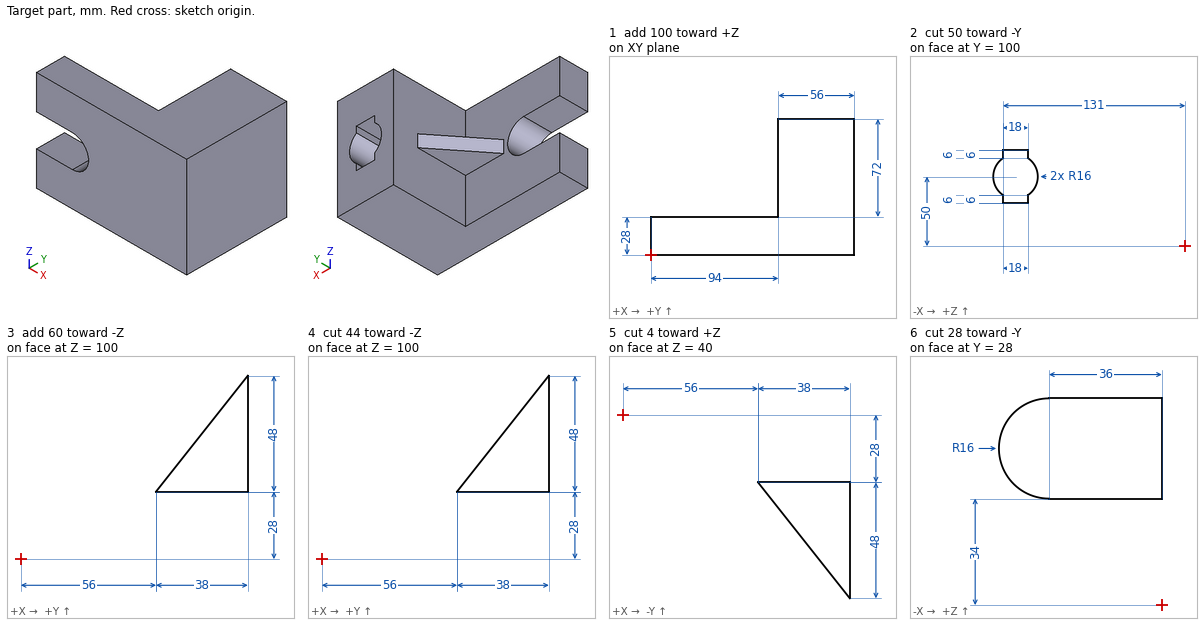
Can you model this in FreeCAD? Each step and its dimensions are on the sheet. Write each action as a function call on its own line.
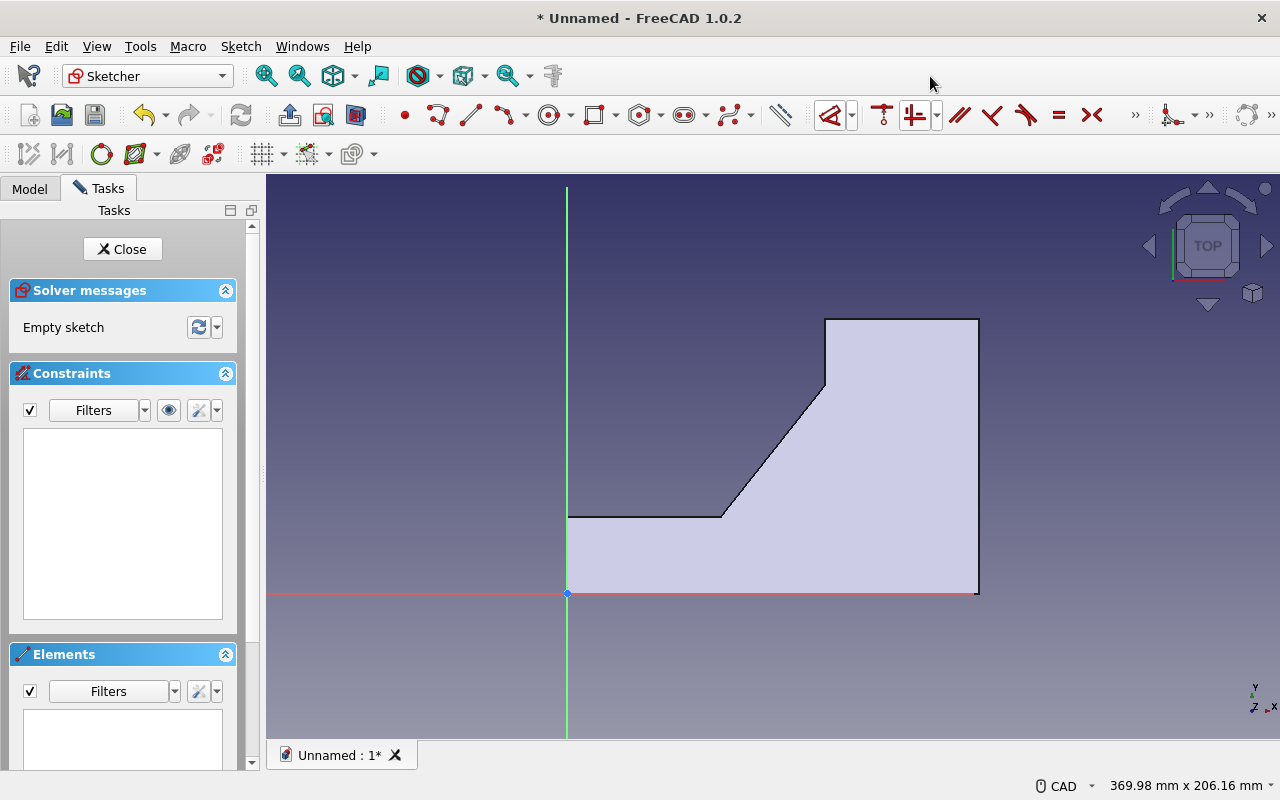
scroll(686, 529, up, 3)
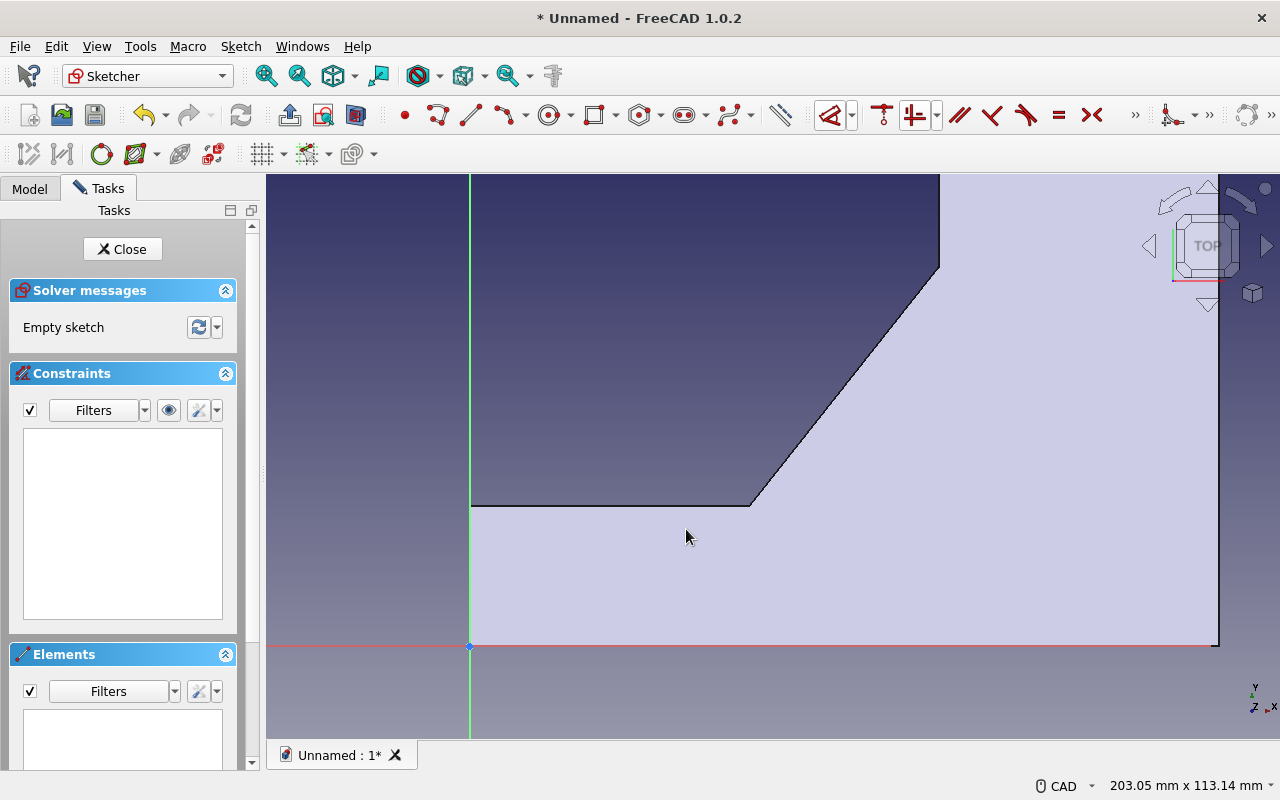
click(438, 116)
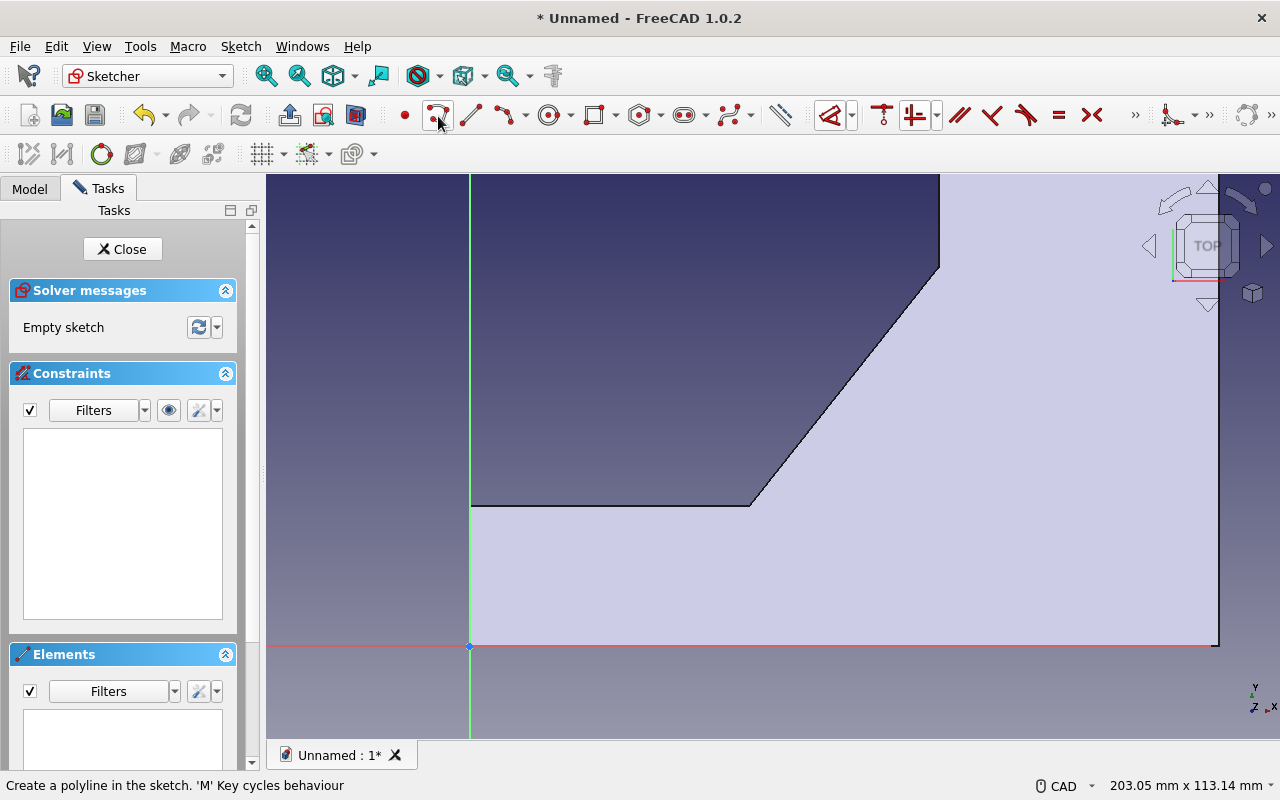
click(749, 506)
click(939, 506)
click(939, 267)
click(749, 507)
key(Escape)
key(Escape)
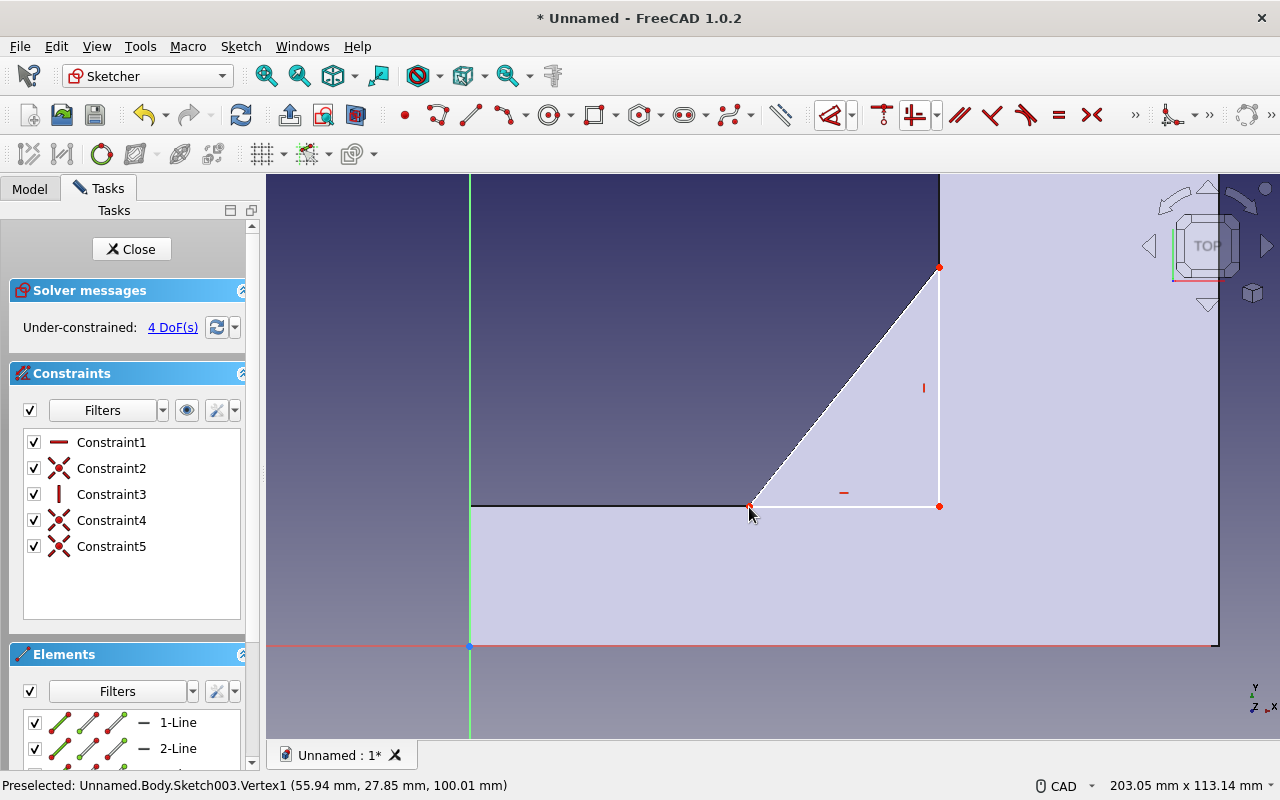
click(806, 507)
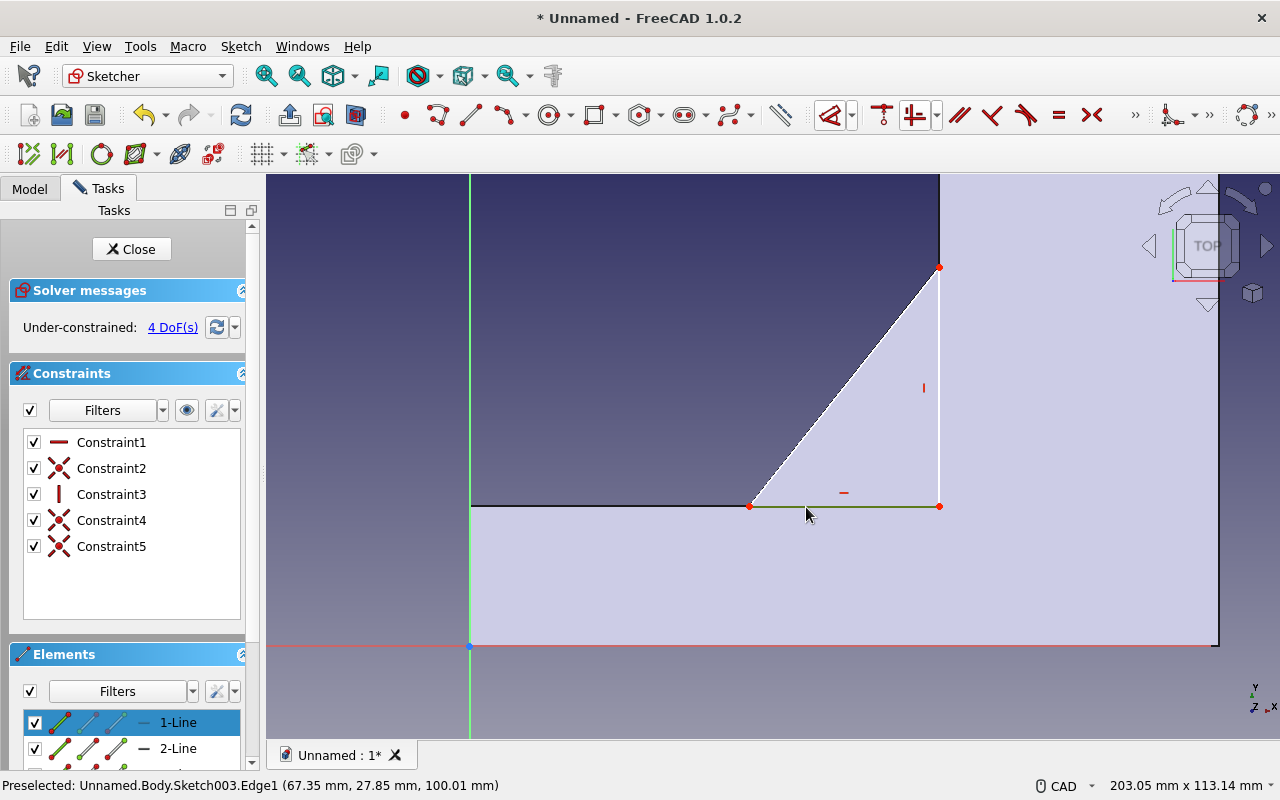
key(l)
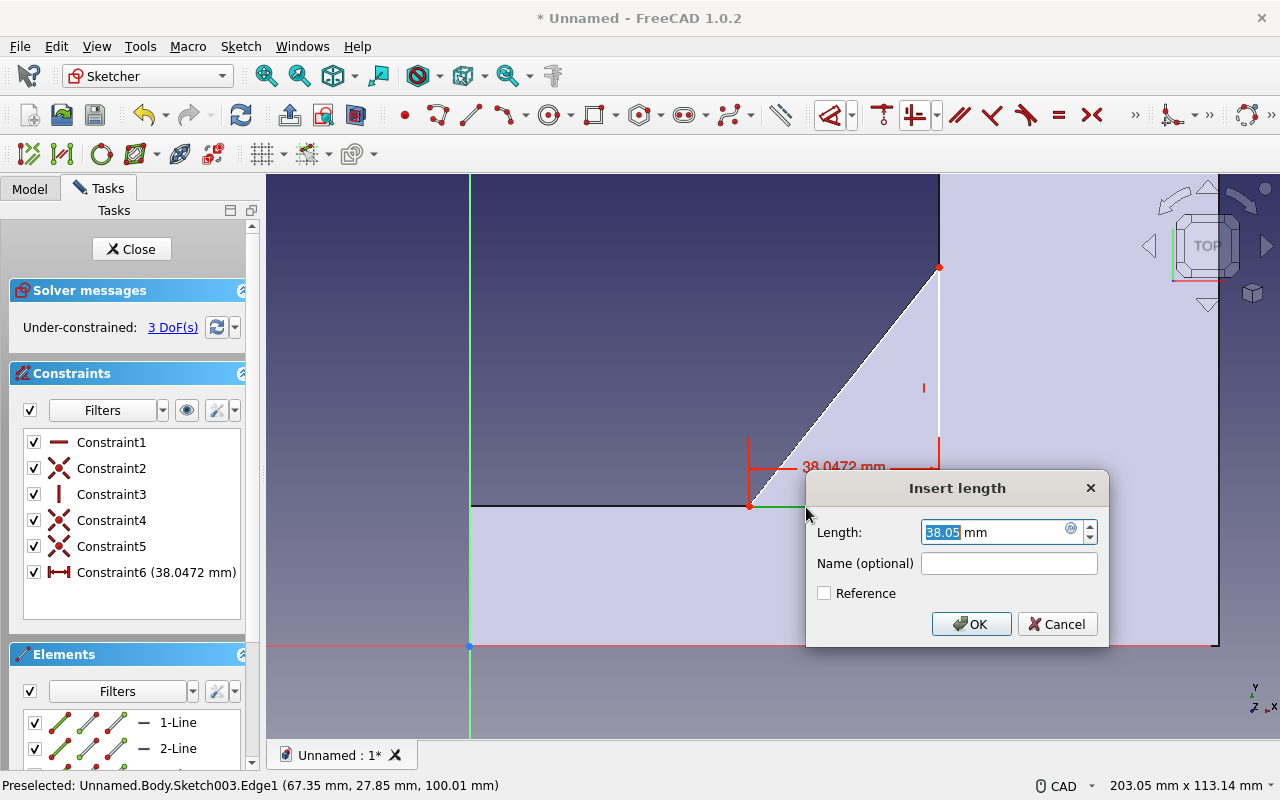
text(38)
key(Return)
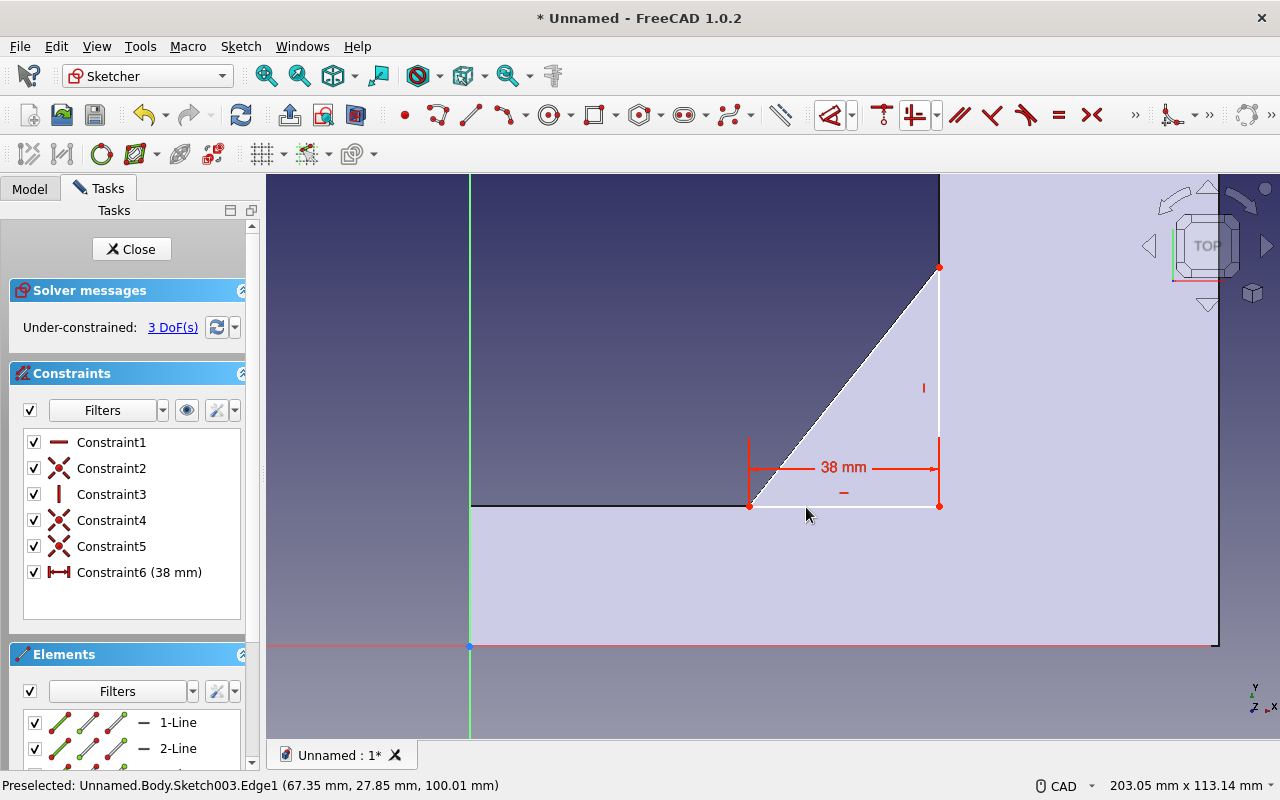
click(939, 435)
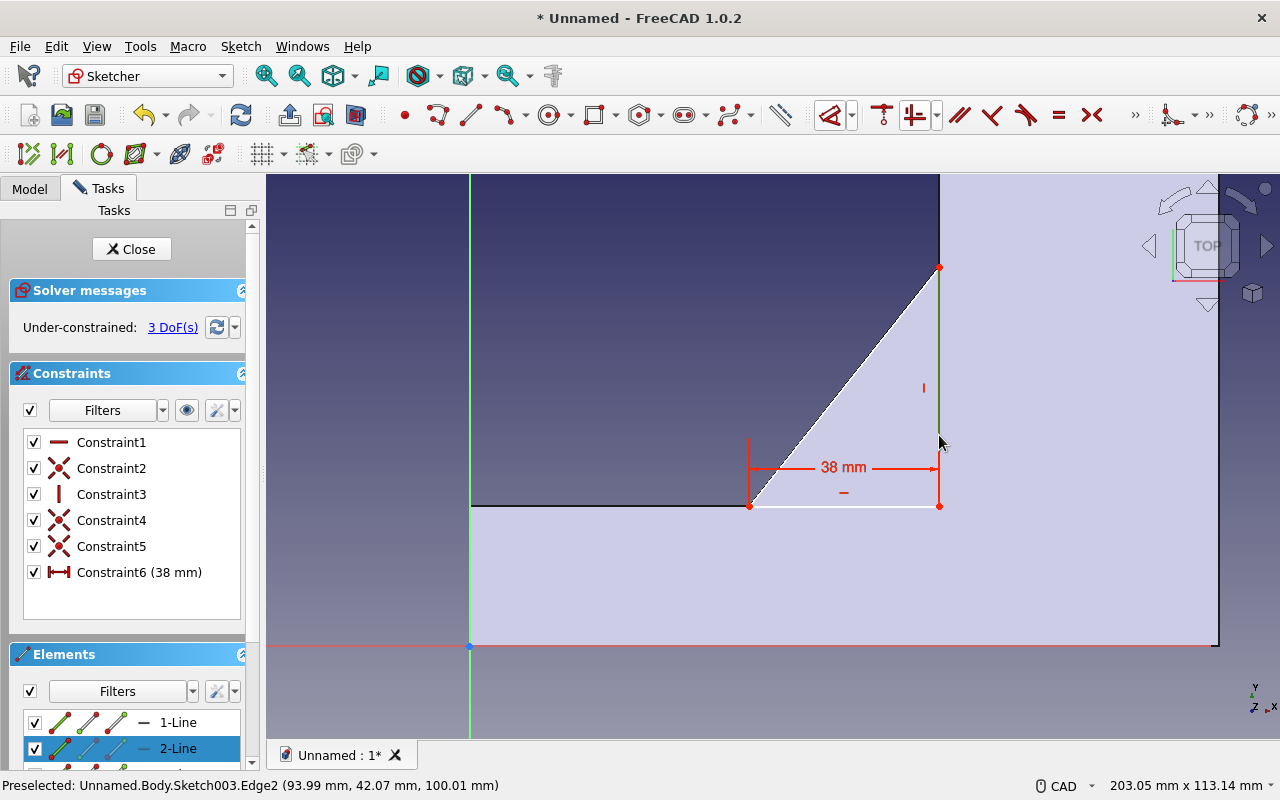
click(852, 116)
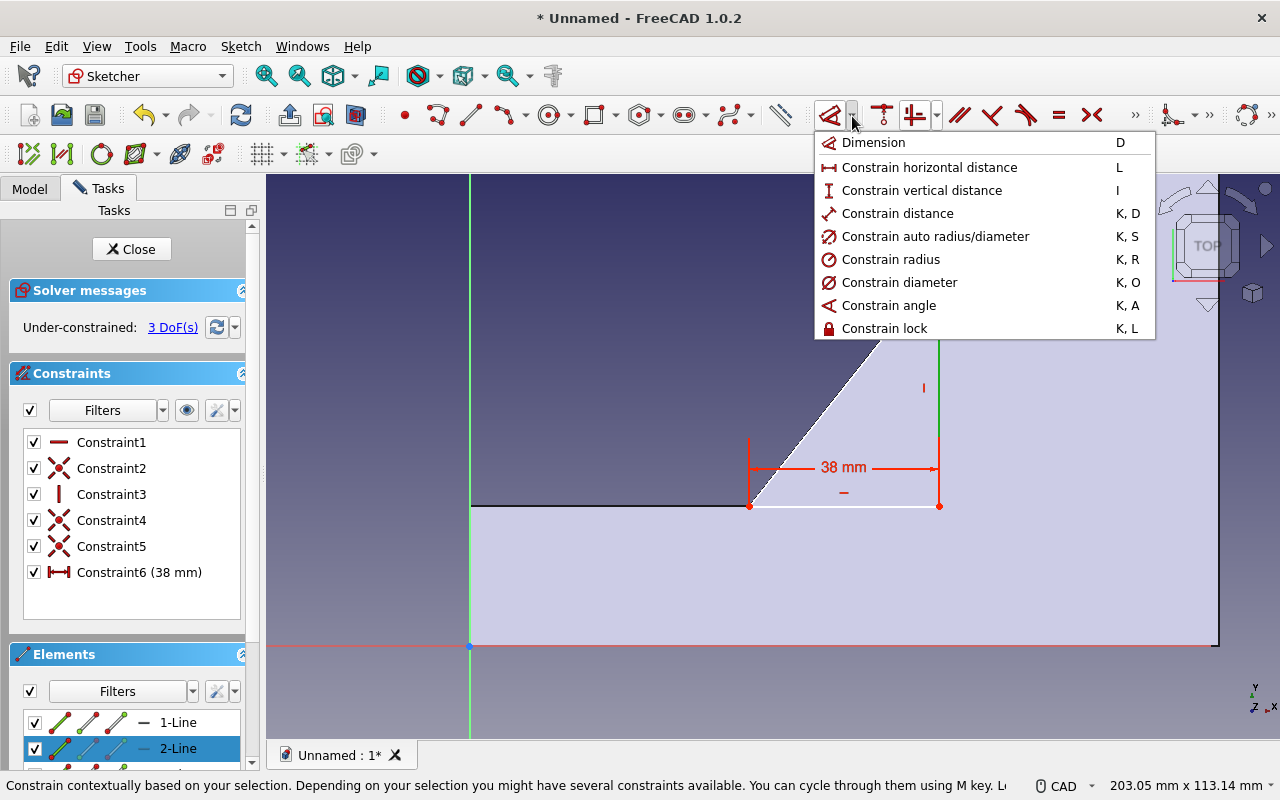
click(985, 190)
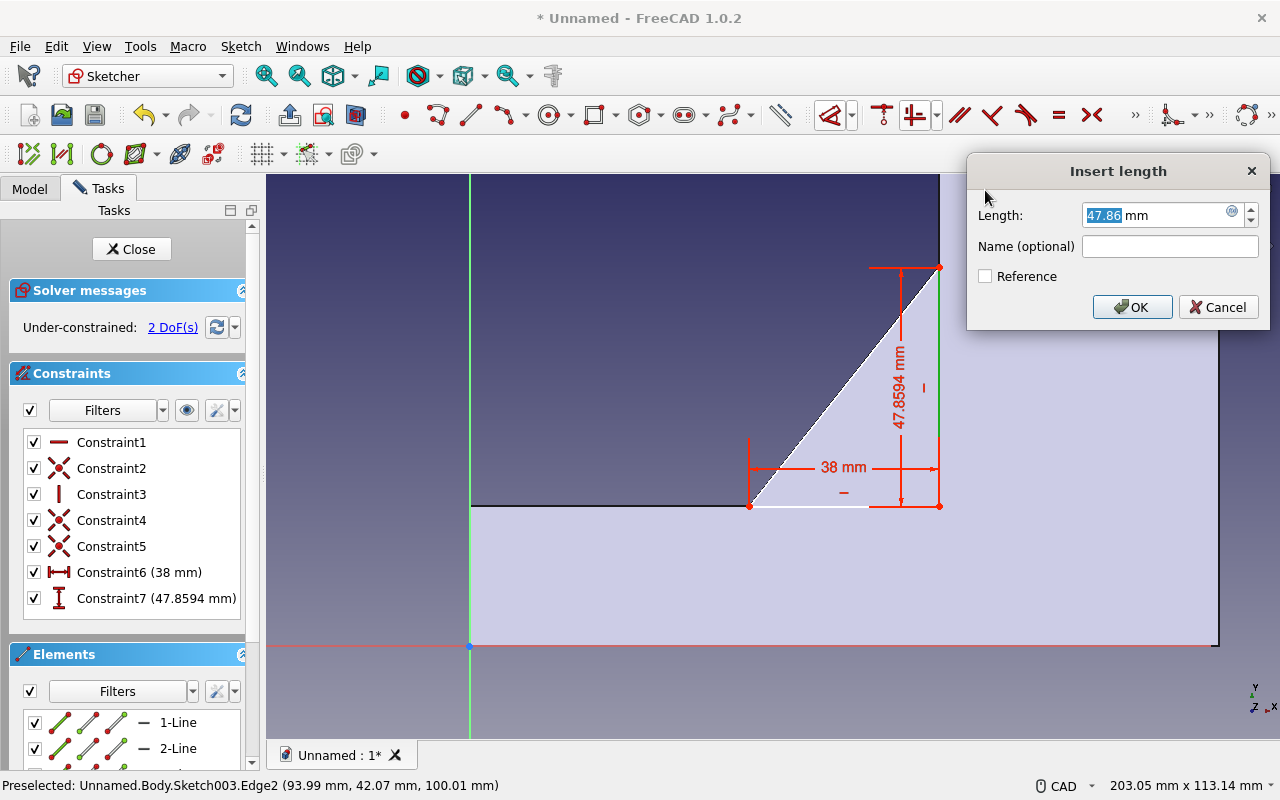
text(48)
key(Return)